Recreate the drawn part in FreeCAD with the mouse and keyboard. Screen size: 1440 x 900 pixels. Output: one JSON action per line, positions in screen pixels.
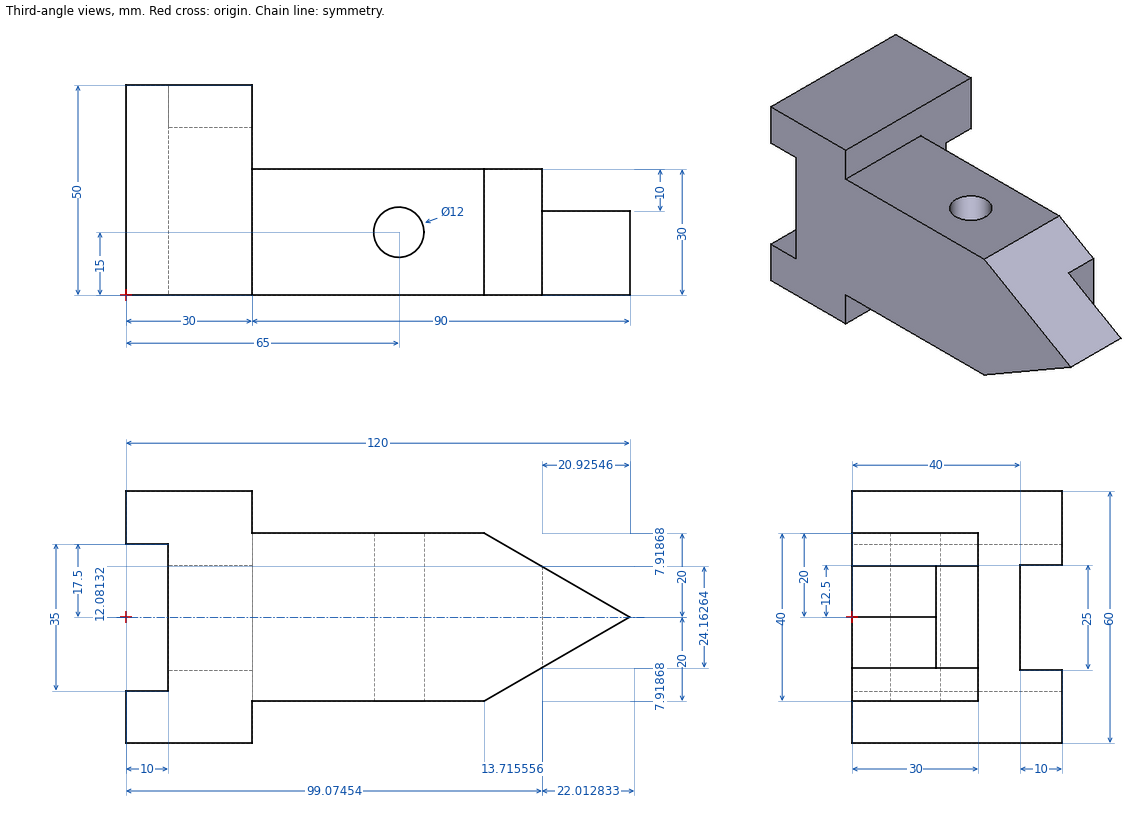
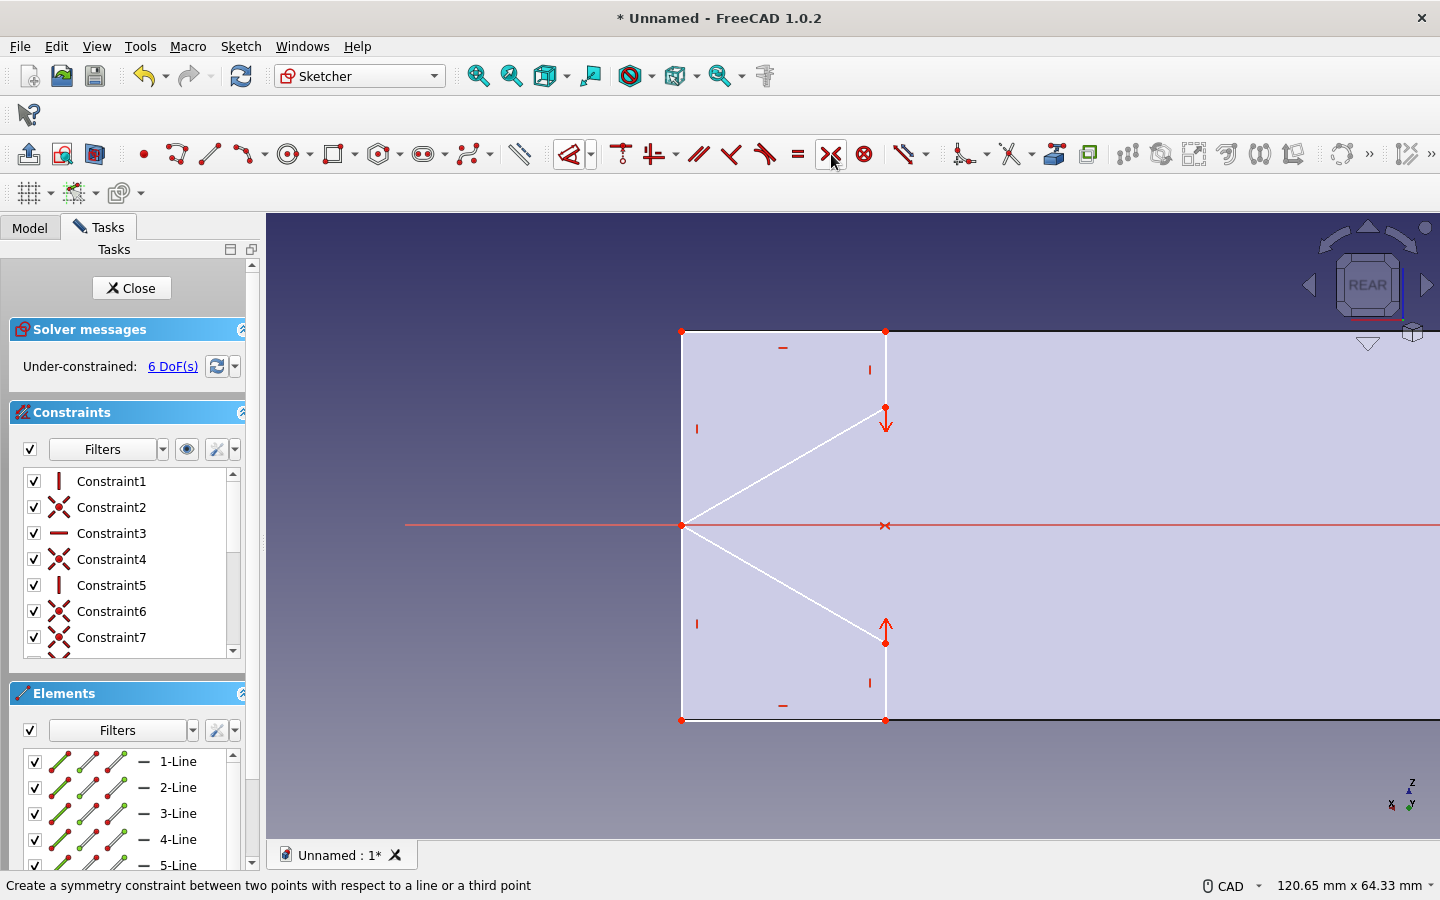
{"action": "left_click", "coordinate": [682, 525]}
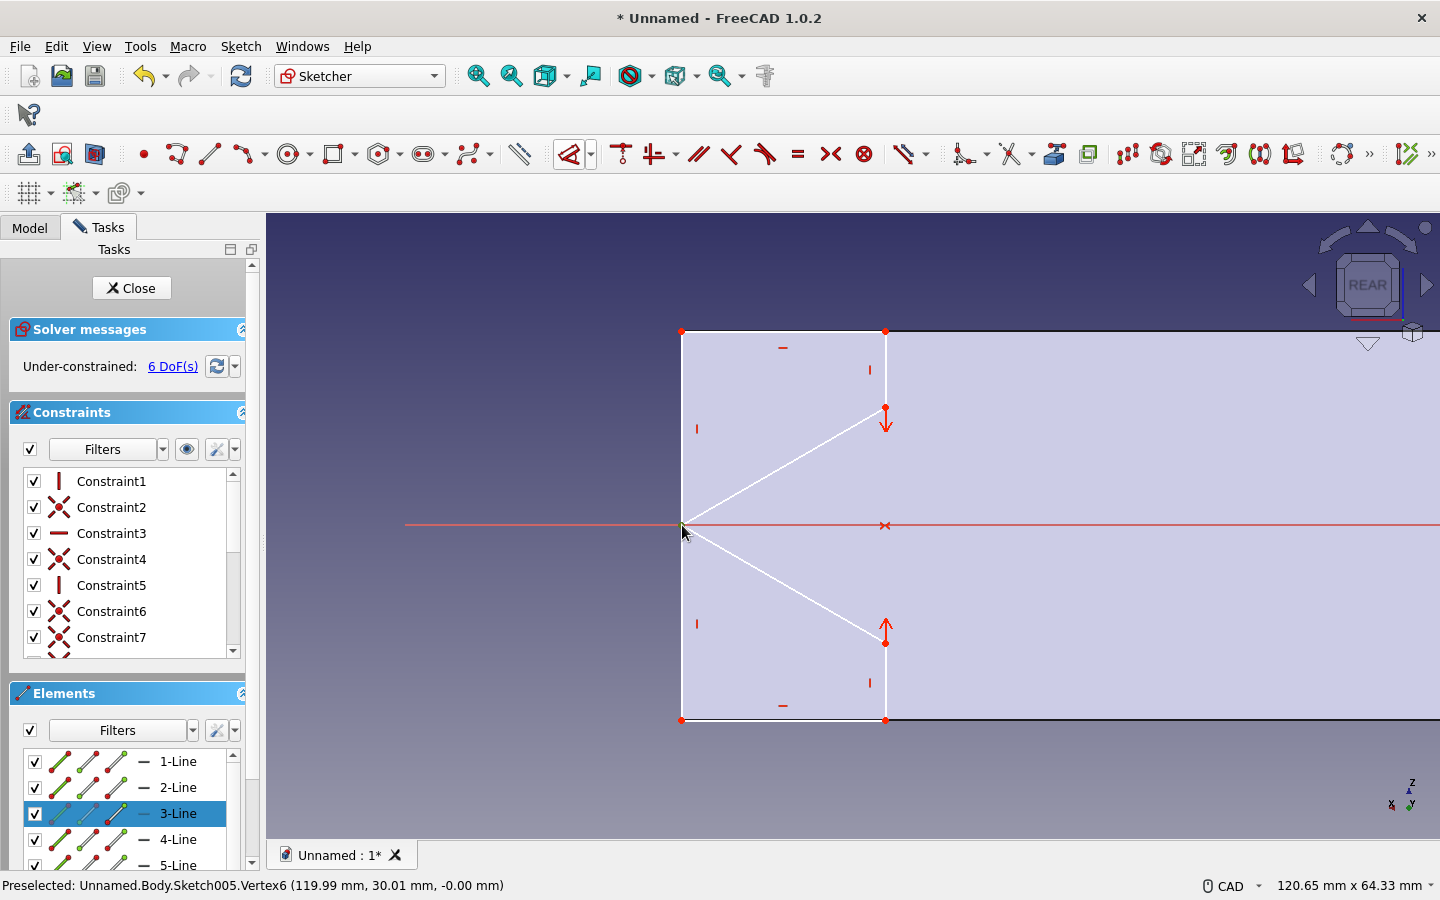
{"action": "left_click", "coordinate": [434, 525]}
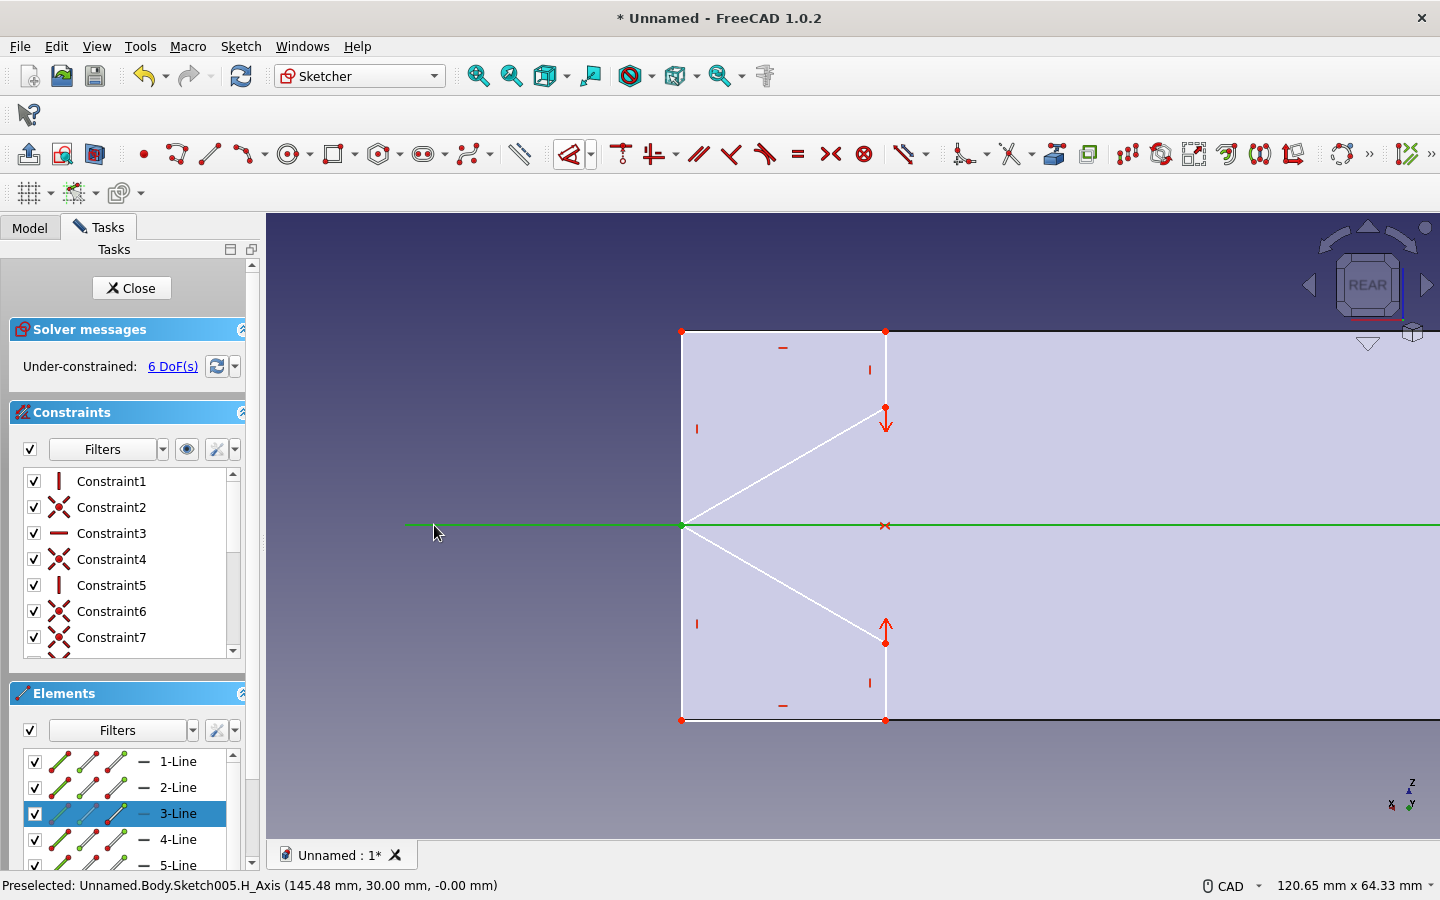
{"action": "left_click", "coordinate": [621, 154]}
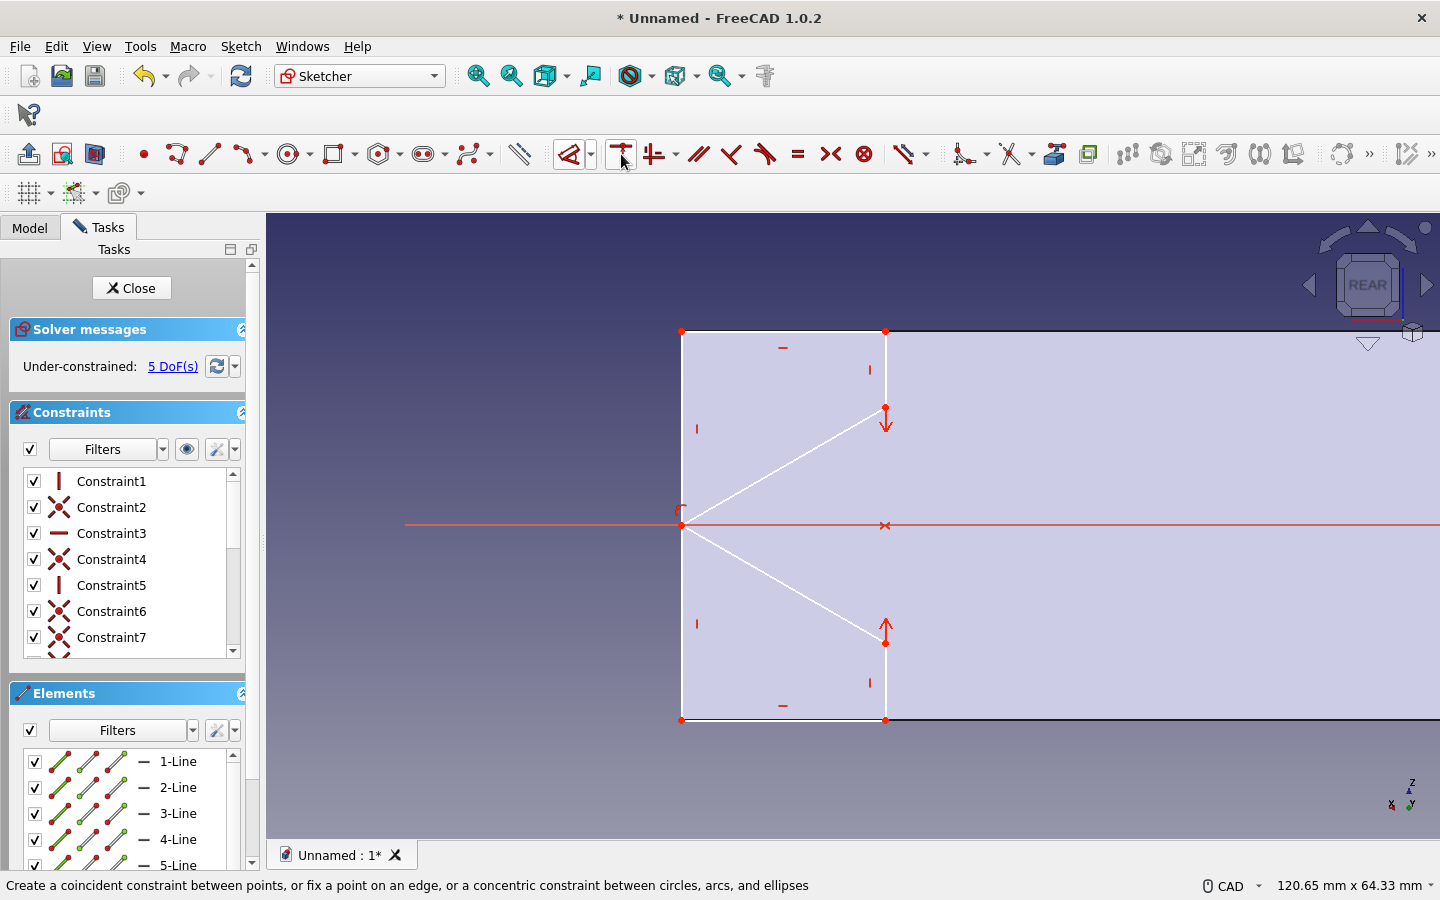
{"action": "left_click", "coordinate": [682, 390]}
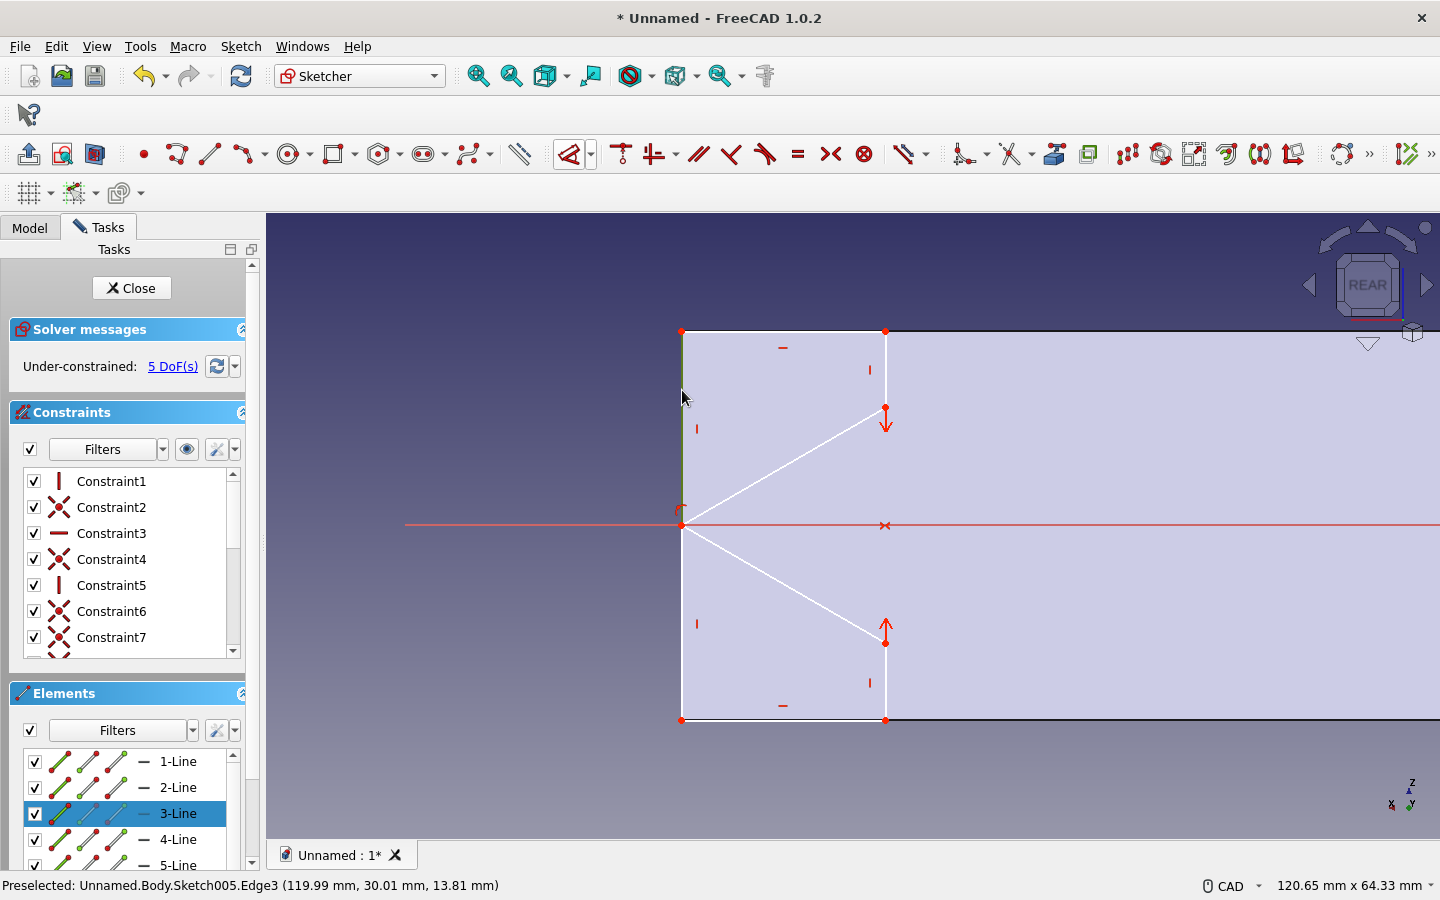
{"action": "key", "text": "i"}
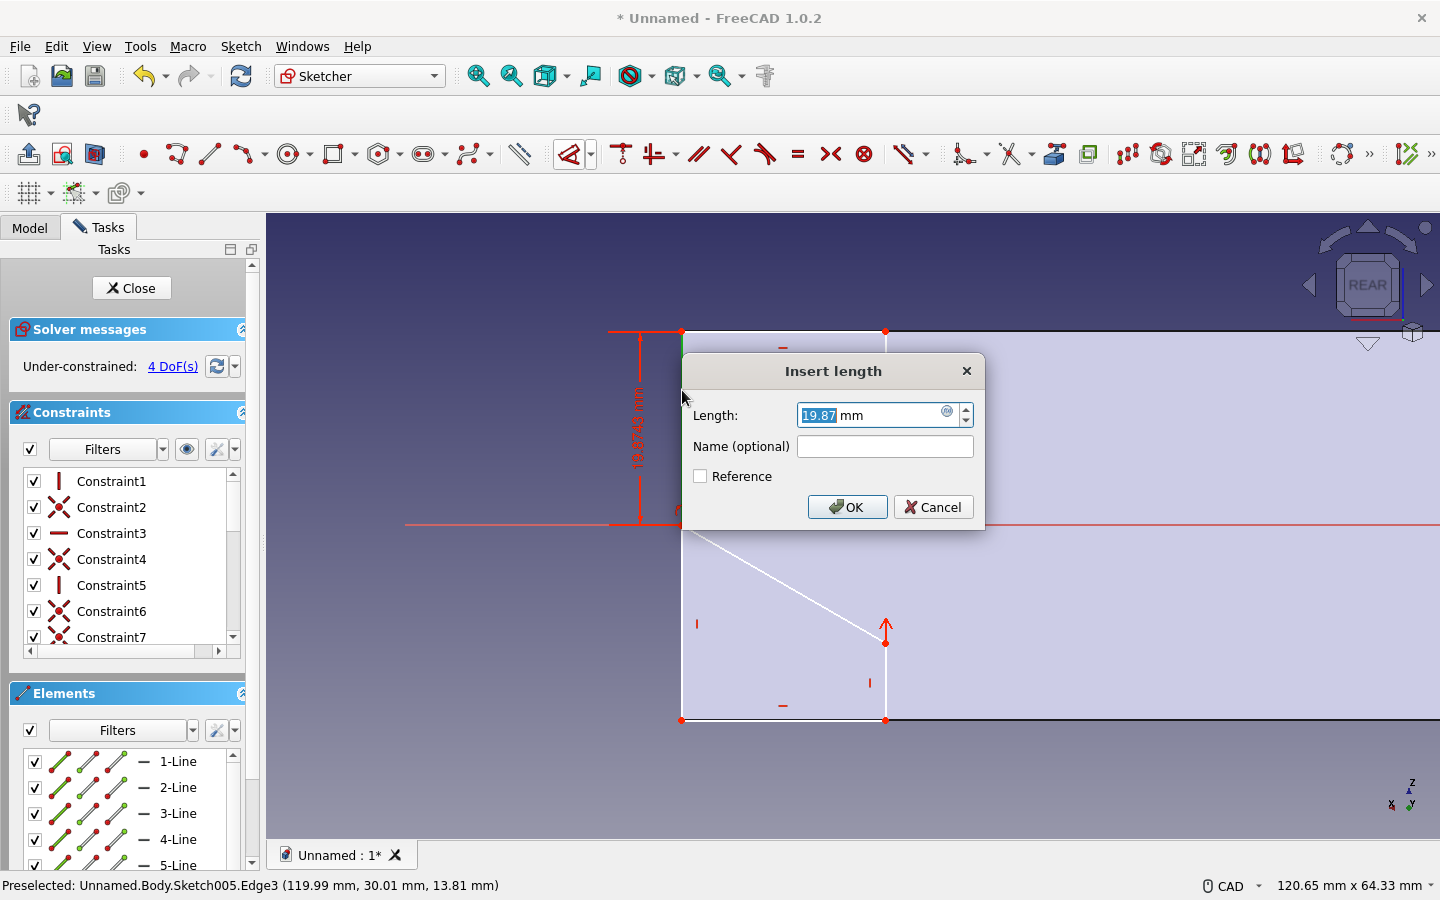
{"action": "type", "text": "20"}
{"action": "key", "text": "Return"}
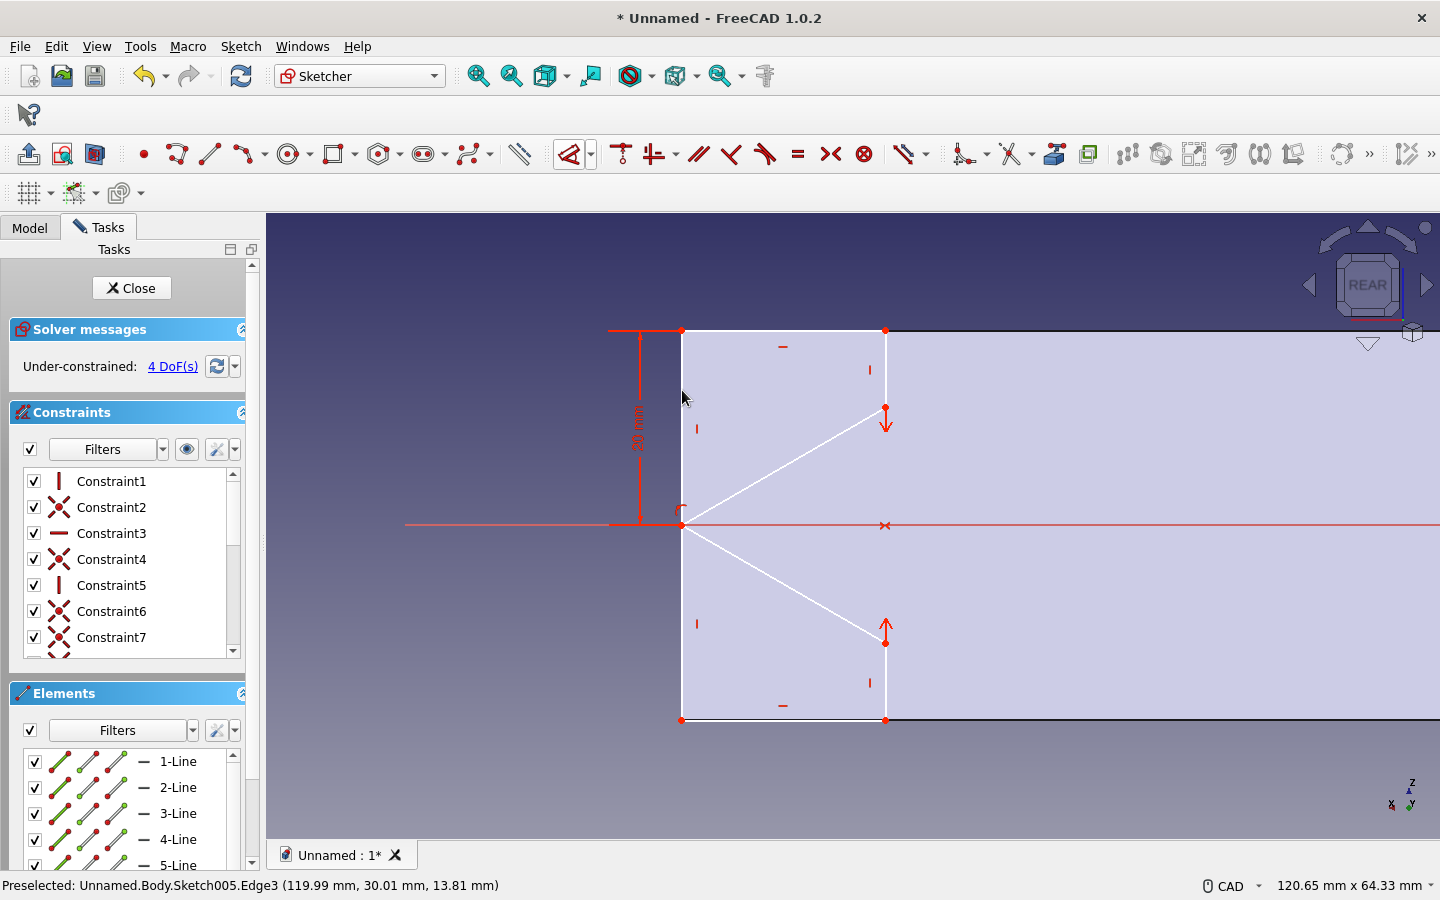
{"action": "left_click", "coordinate": [682, 584]}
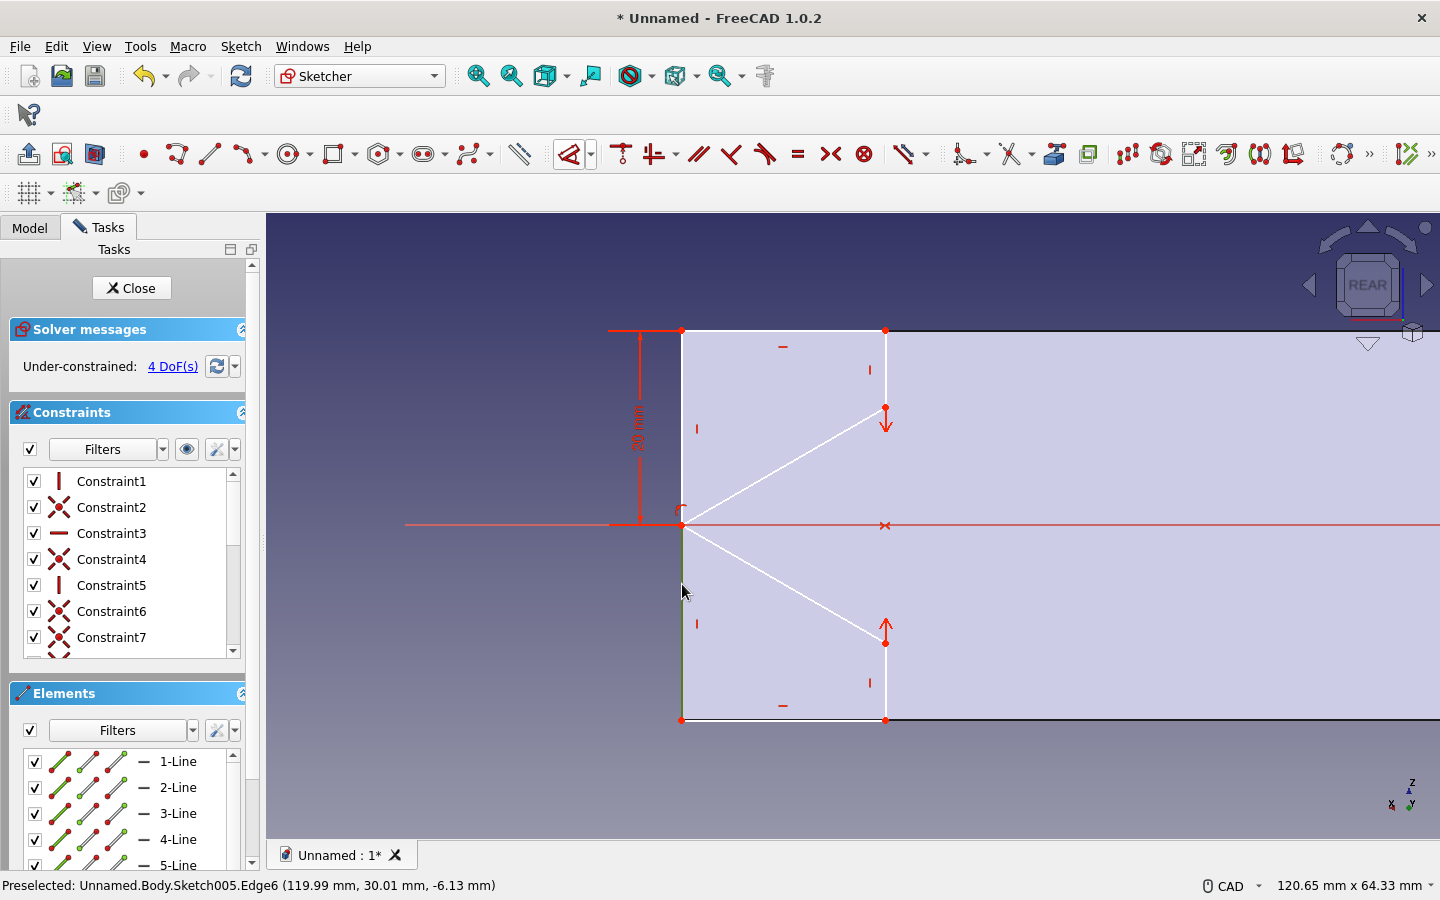
{"action": "left_click", "coordinate": [590, 154]}